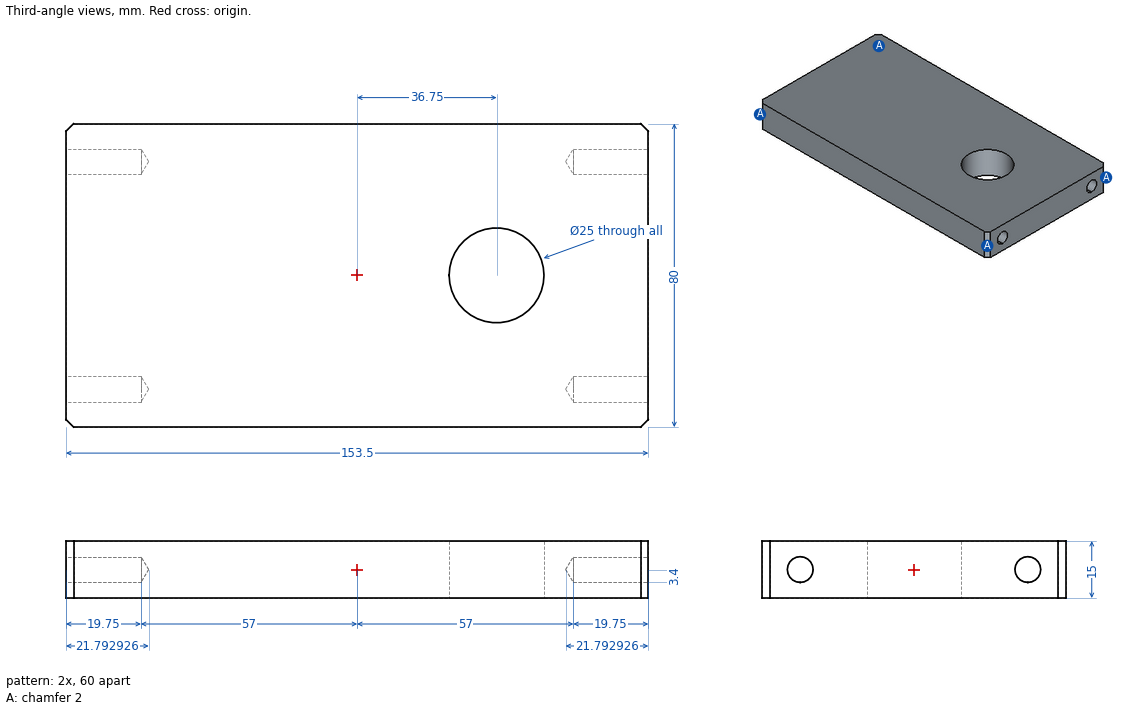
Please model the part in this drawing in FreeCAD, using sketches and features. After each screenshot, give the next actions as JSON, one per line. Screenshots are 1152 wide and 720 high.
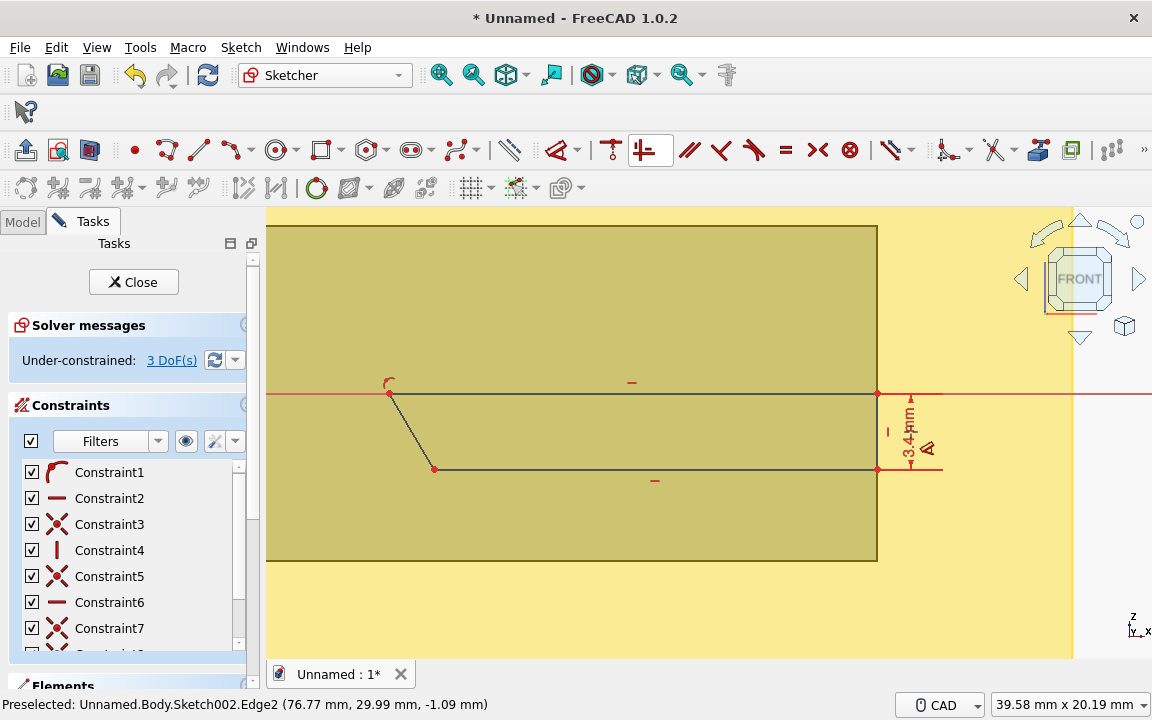
{"action": "left_click", "coordinate": [434, 470]}
{"action": "left_click", "coordinate": [364, 504]}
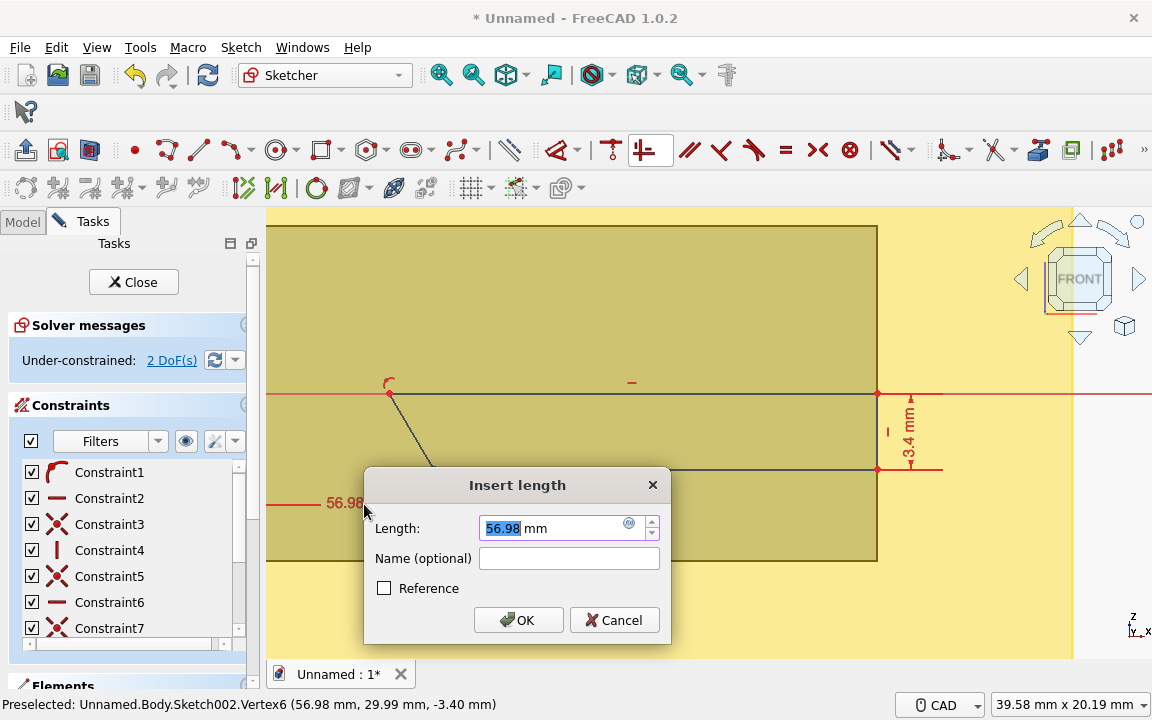
{"action": "type", "text": "57"}
{"action": "key", "text": "Return"}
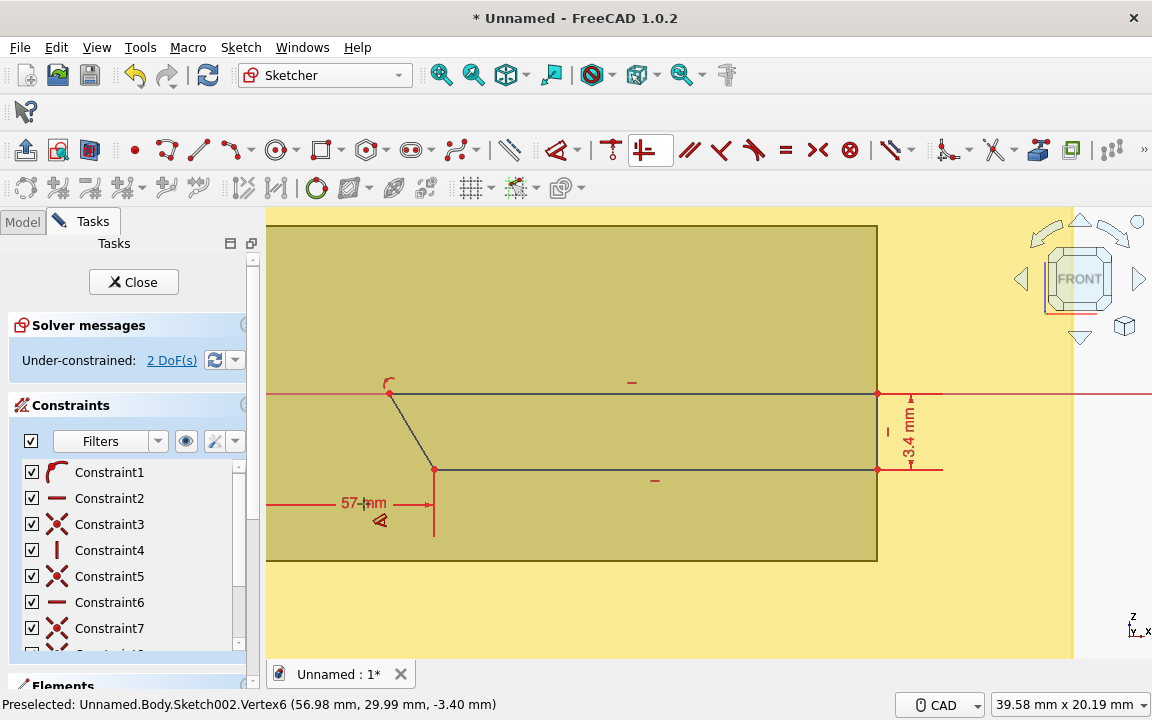
{"action": "left_click", "coordinate": [744, 470]}
{"action": "left_click", "coordinate": [656, 504]}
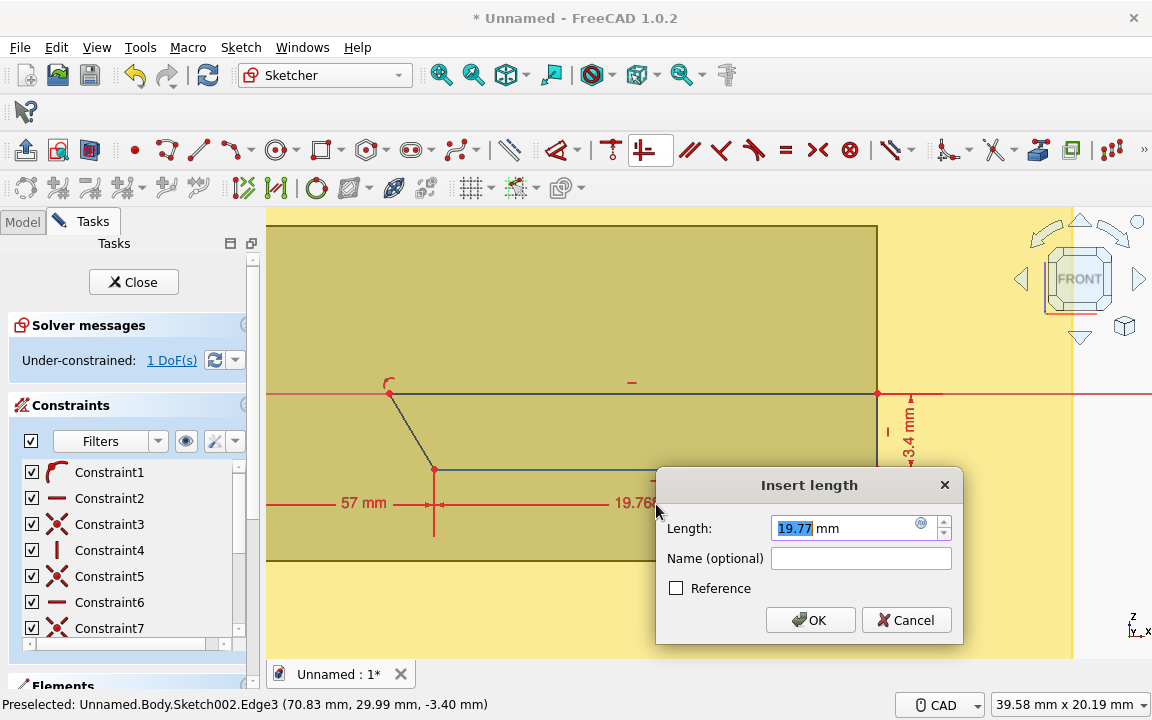
{"action": "type", "text": "19.75"}
{"action": "key", "text": "Return"}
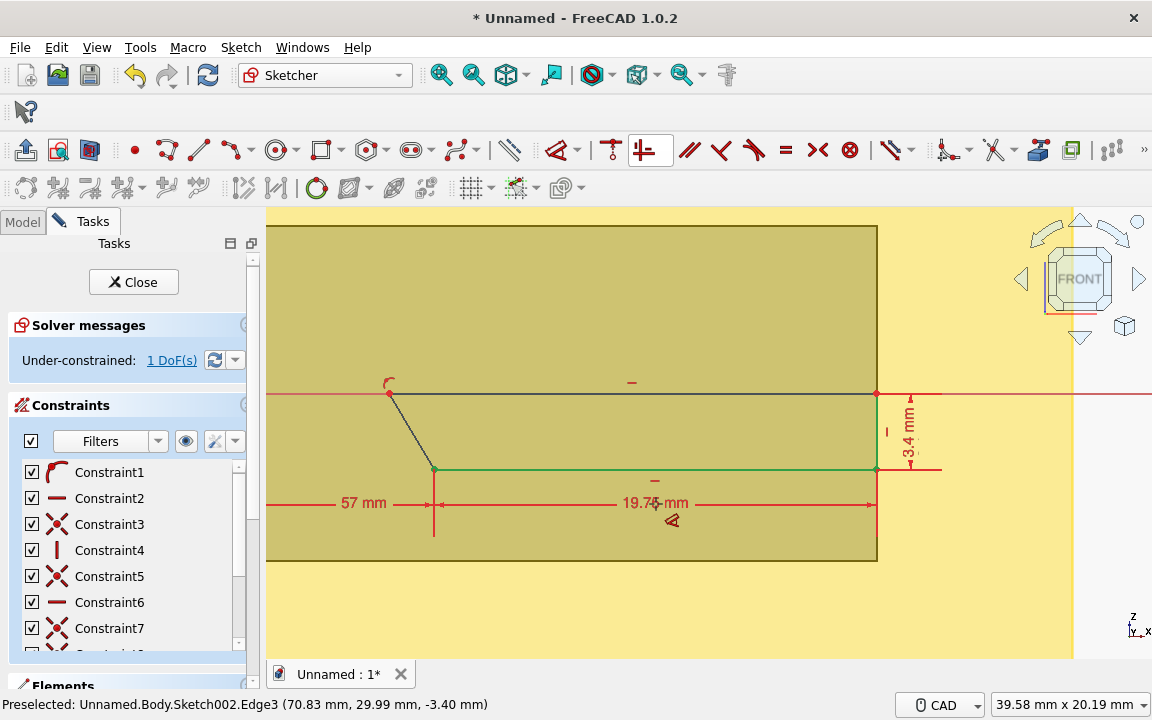
{"action": "left_click", "coordinate": [535, 394]}
{"action": "left_click", "coordinate": [633, 360]}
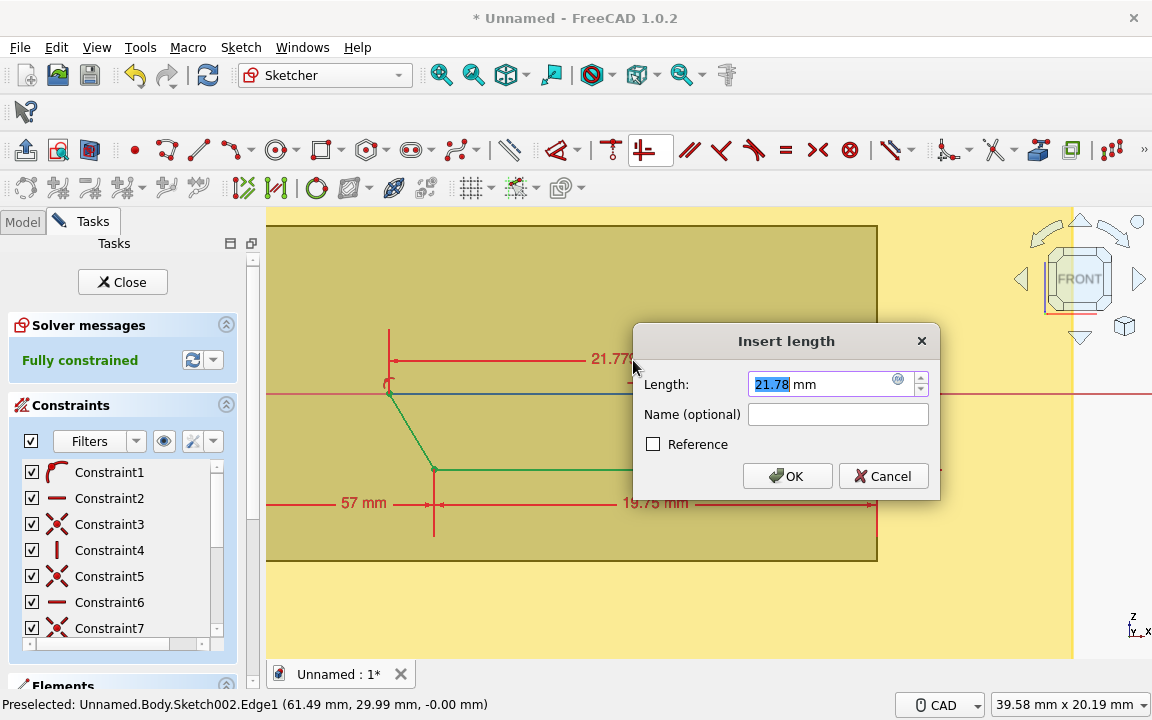
{"action": "type", "text": "21.792926"}
{"action": "key", "text": "Return"}
{"action": "key", "text": "Escape"}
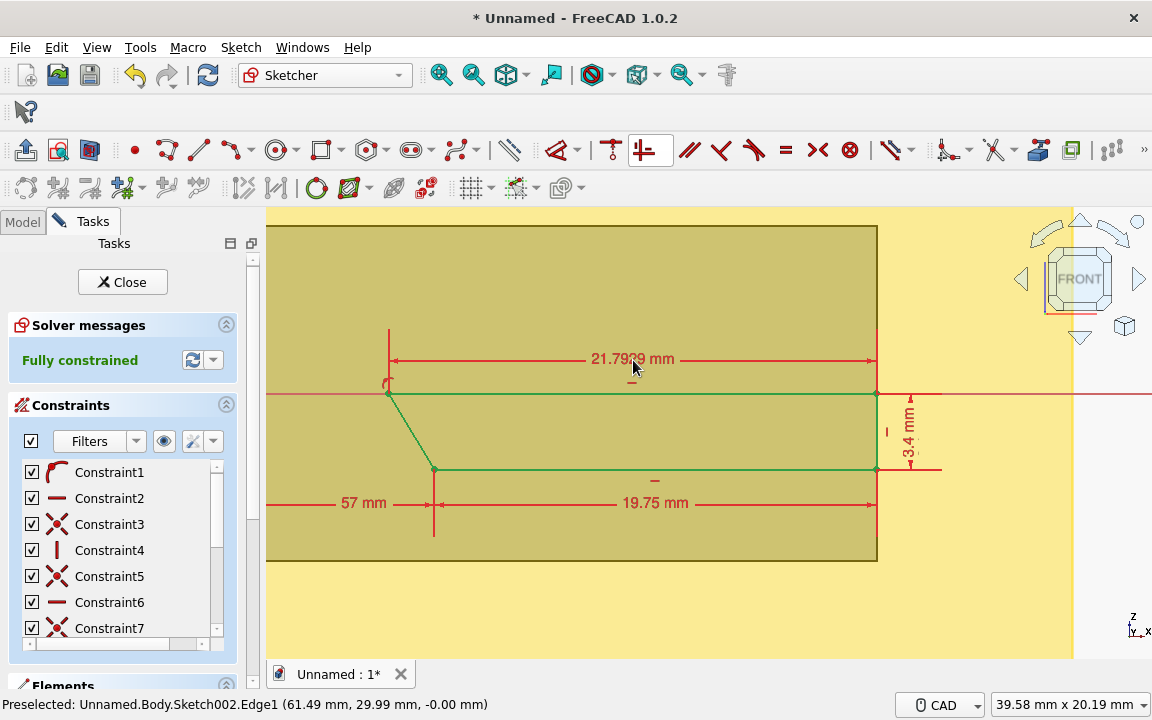
{"action": "left_click", "coordinate": [123, 282]}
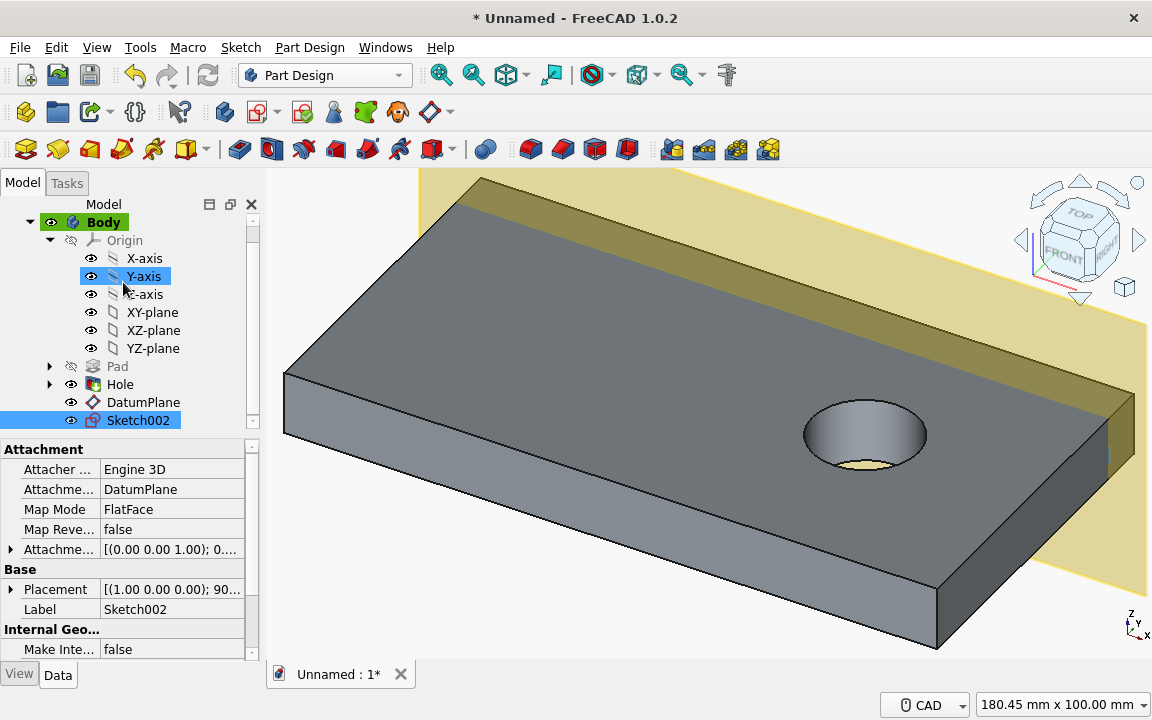
{"action": "left_click", "coordinate": [304, 150]}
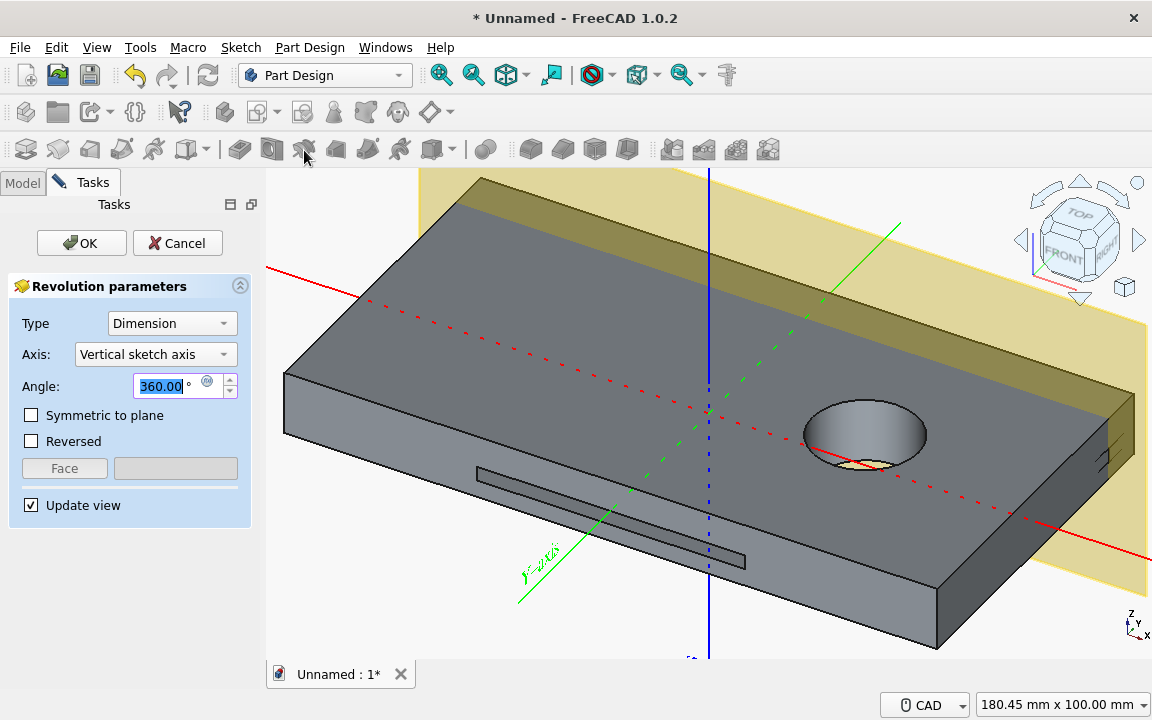
{"action": "left_click", "coordinate": [156, 354]}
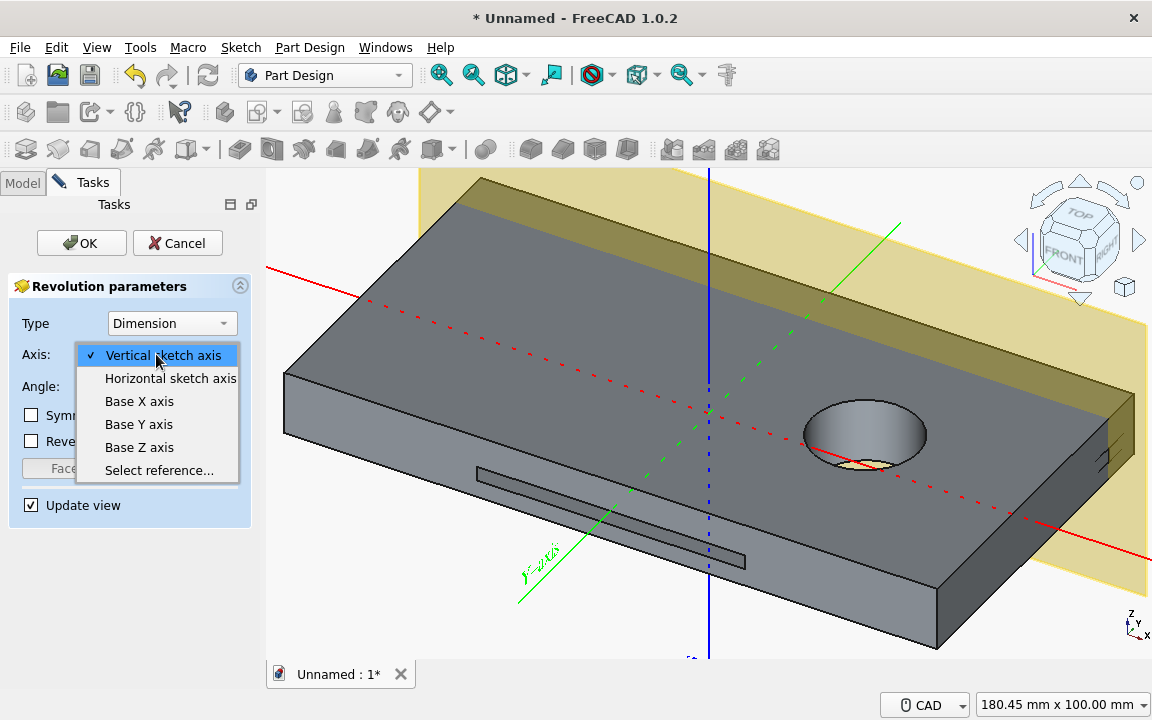
{"action": "left_click", "coordinate": [156, 378]}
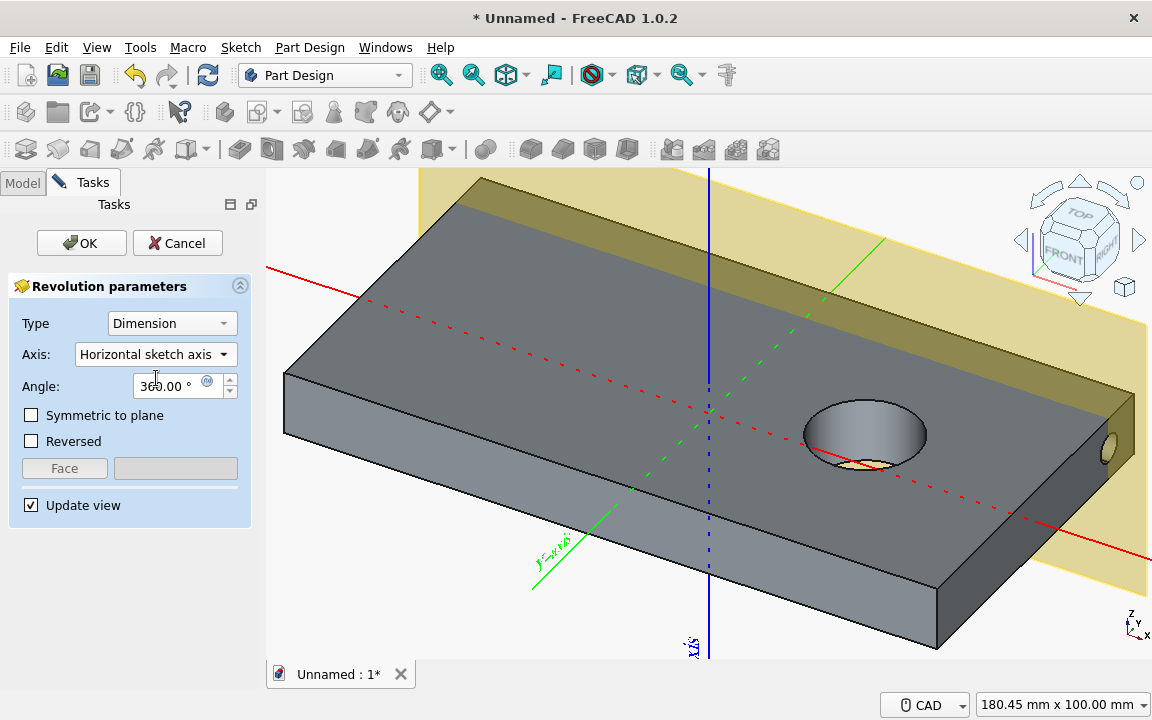
{"action": "left_click", "coordinate": [82, 243]}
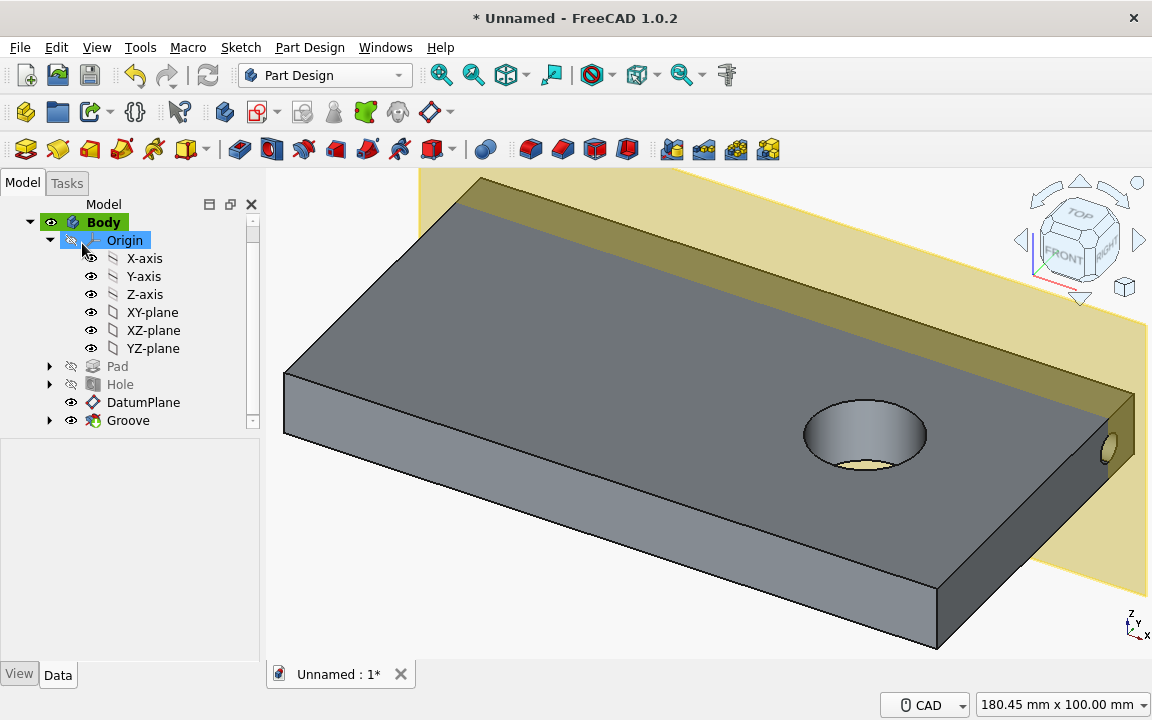
{"action": "left_click", "coordinate": [116, 402]}
{"action": "key", "text": "space"}